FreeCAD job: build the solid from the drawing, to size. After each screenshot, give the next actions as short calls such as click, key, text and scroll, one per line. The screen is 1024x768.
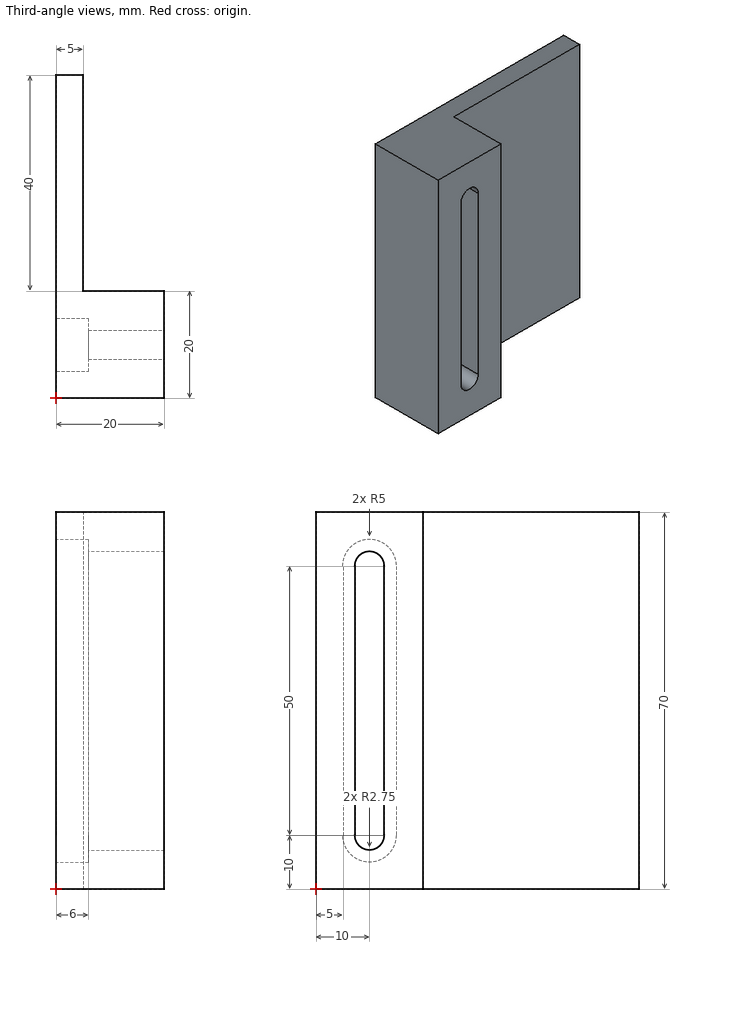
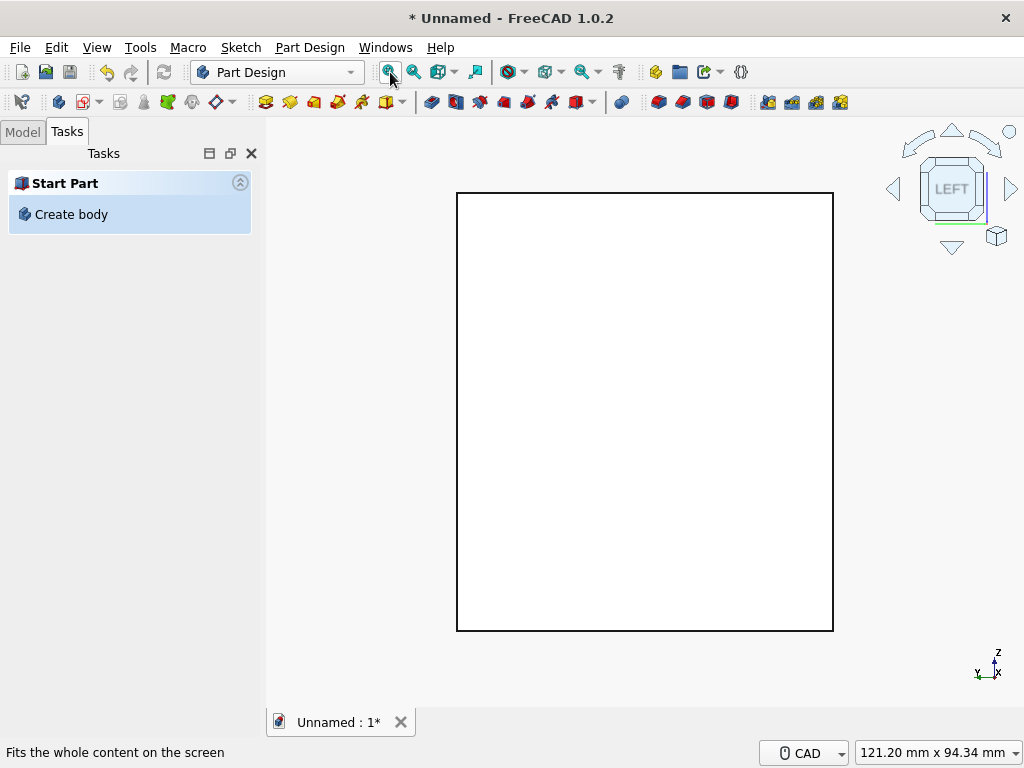
click(645, 411)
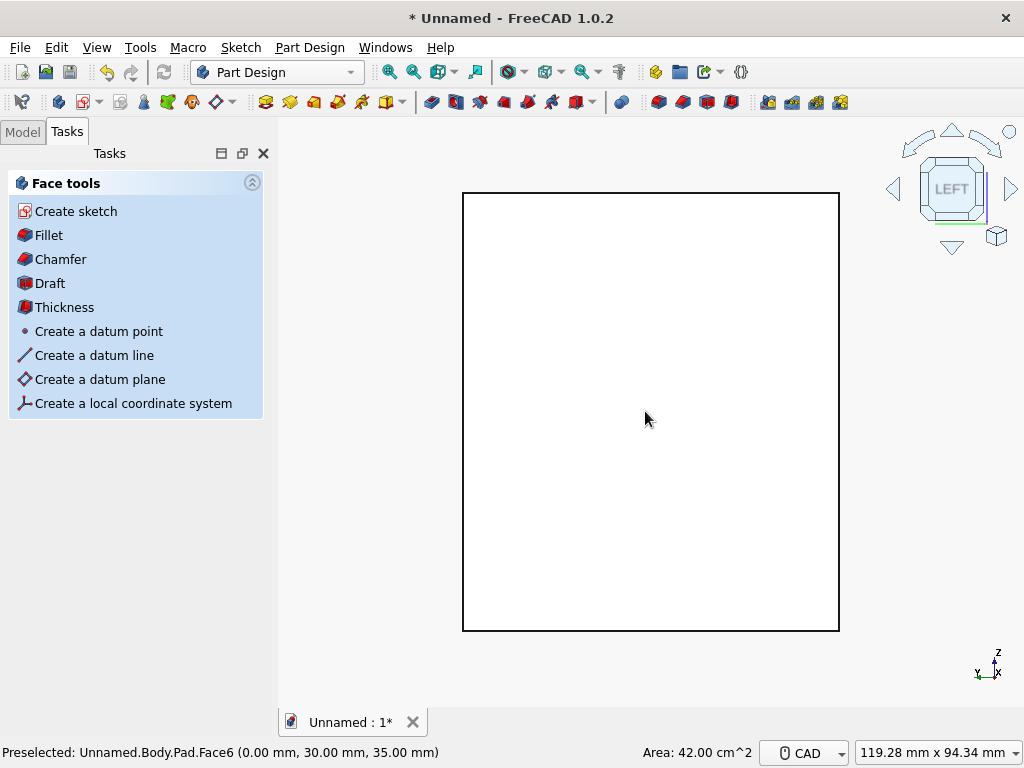
click(84, 102)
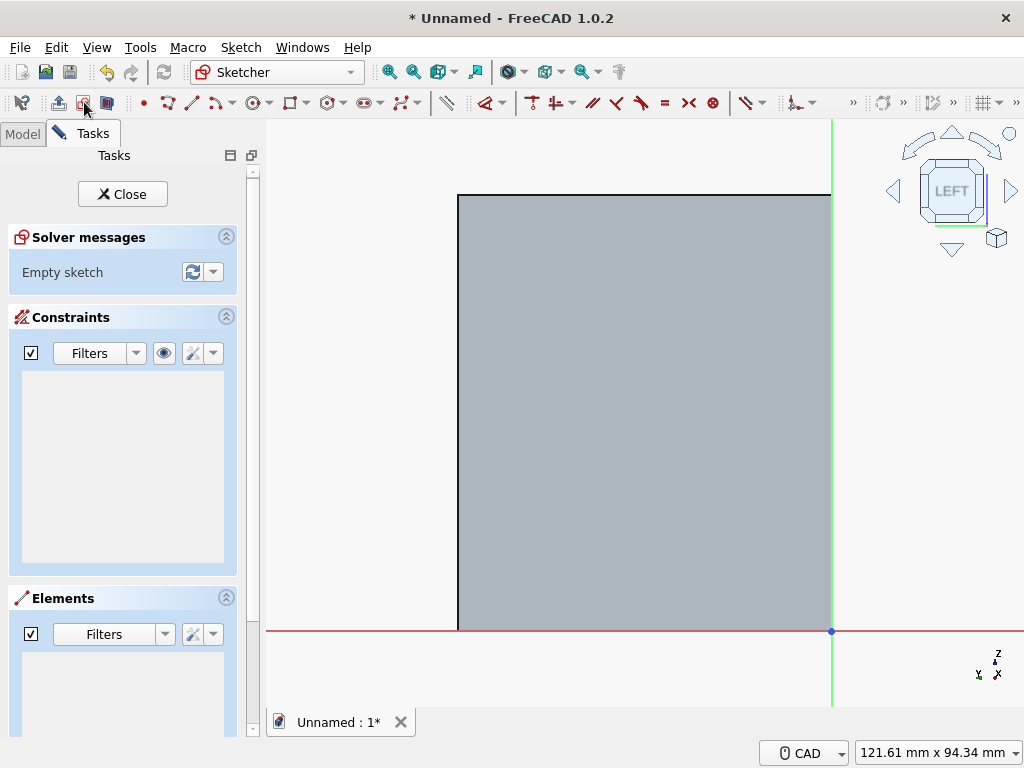
click(364, 104)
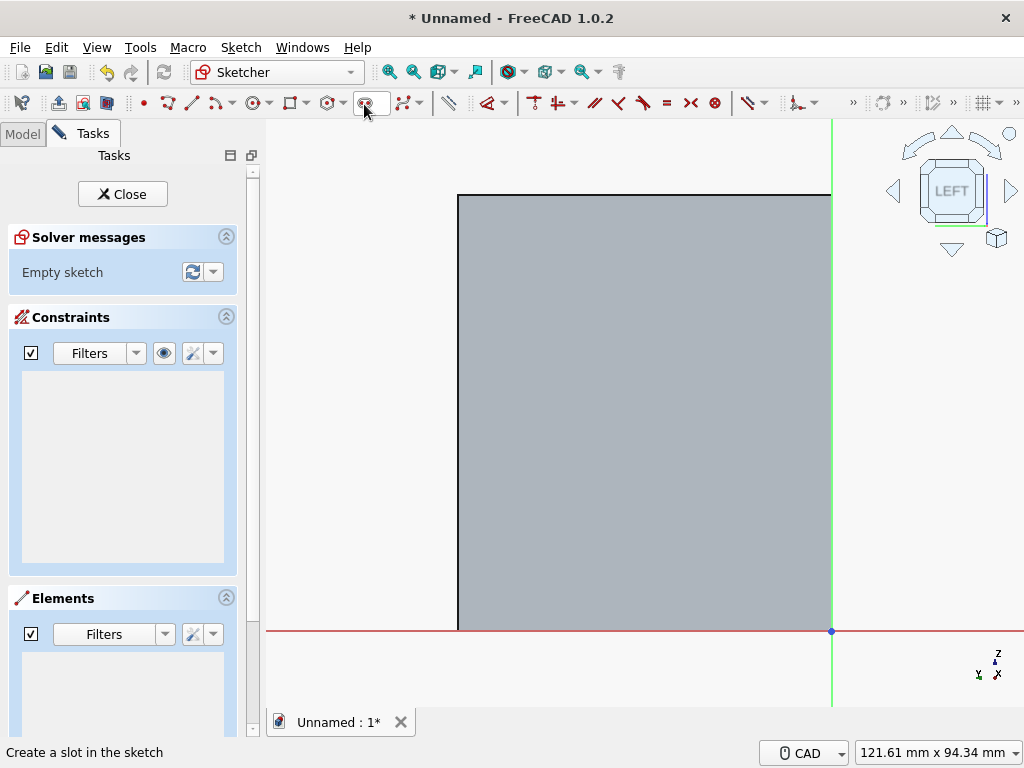
scroll(770, 569, up, 2)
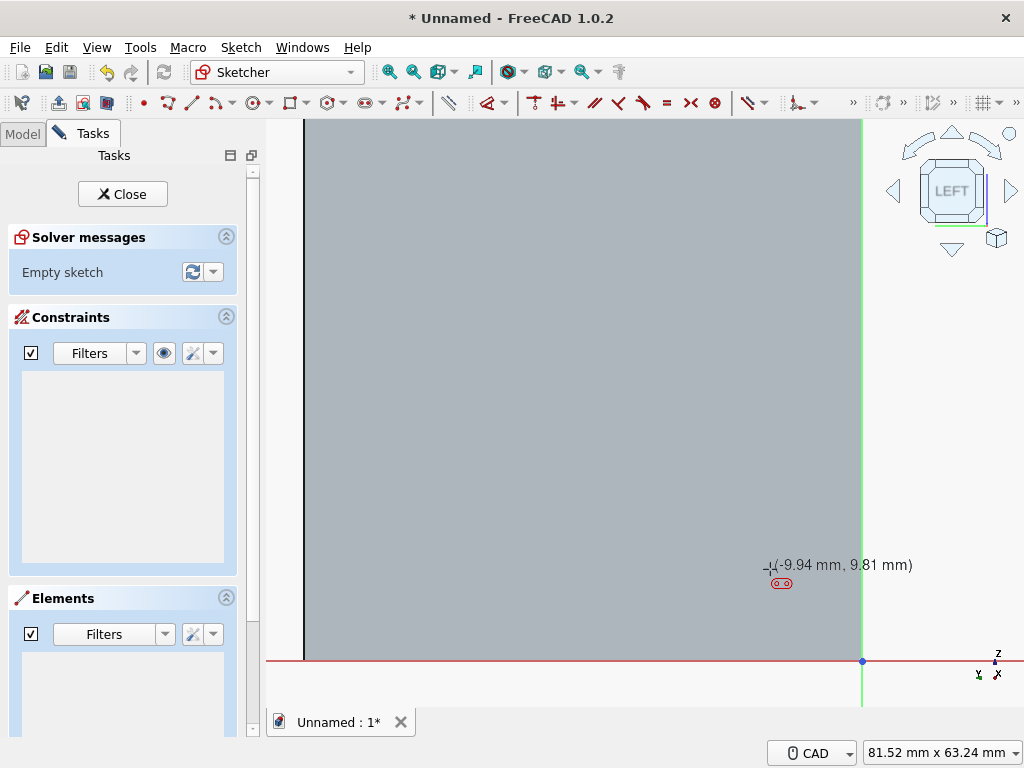
click(769, 568)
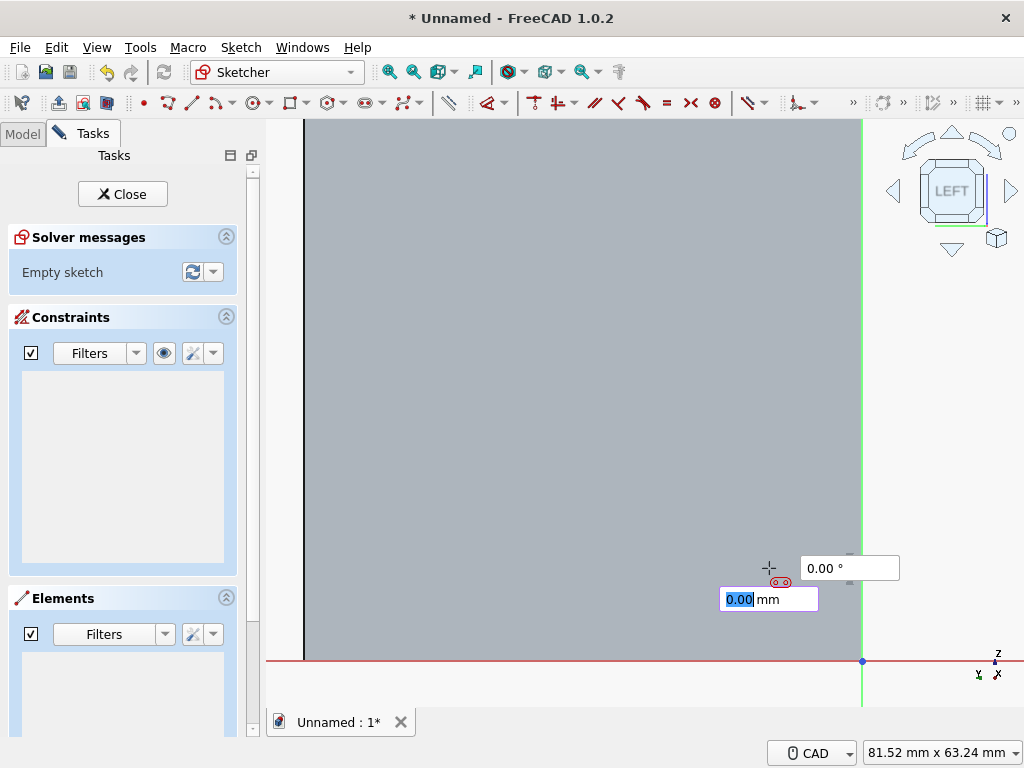
scroll(294, 501, down, 2)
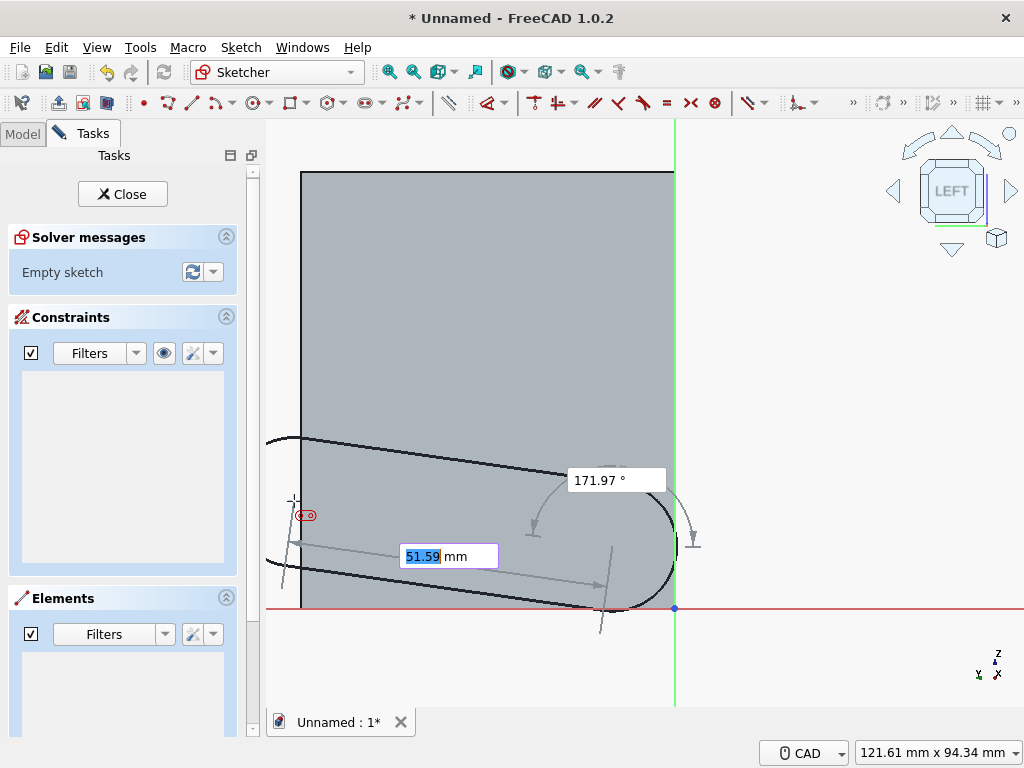
click(612, 235)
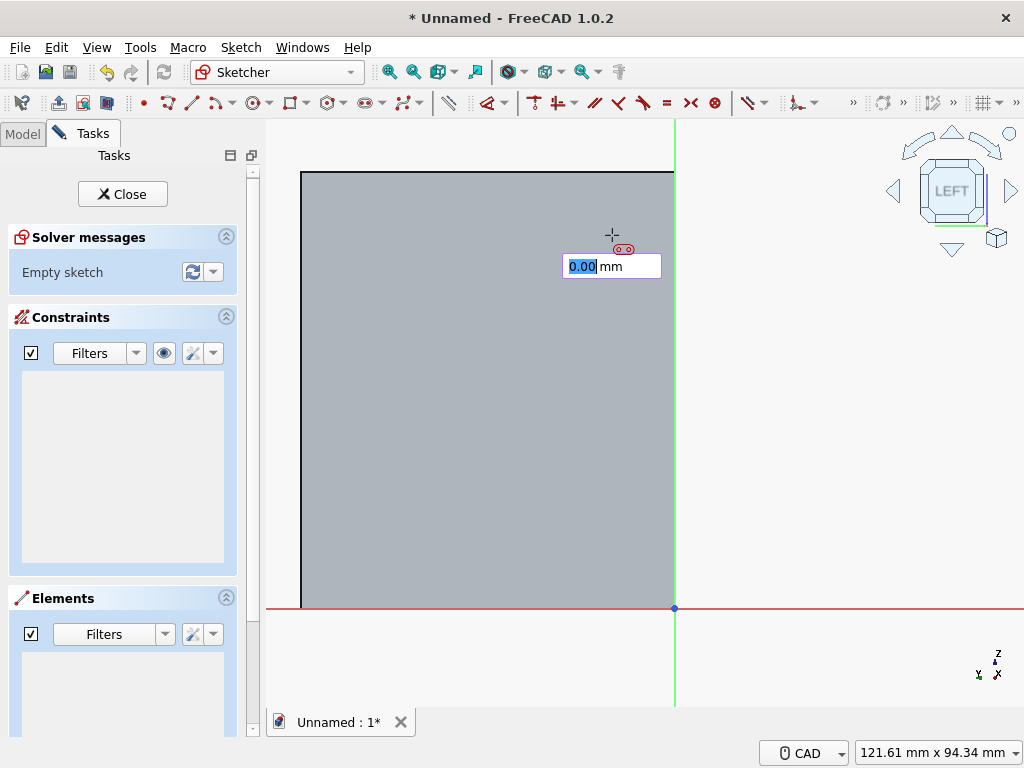
click(595, 391)
key(Escape)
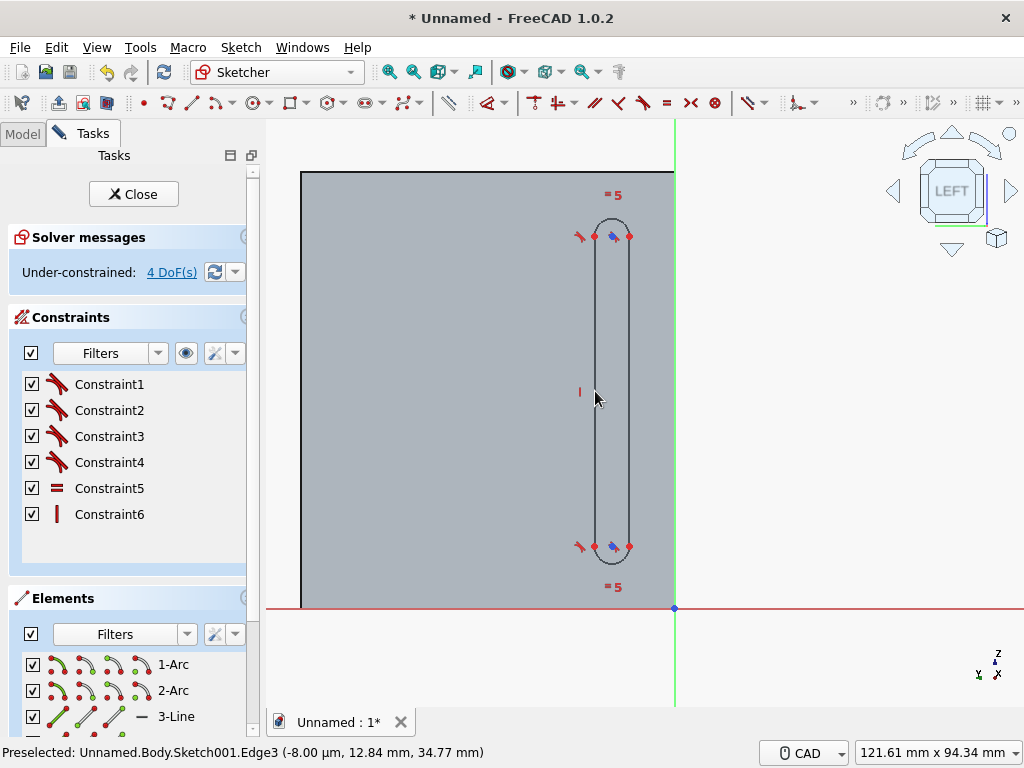
click(488, 104)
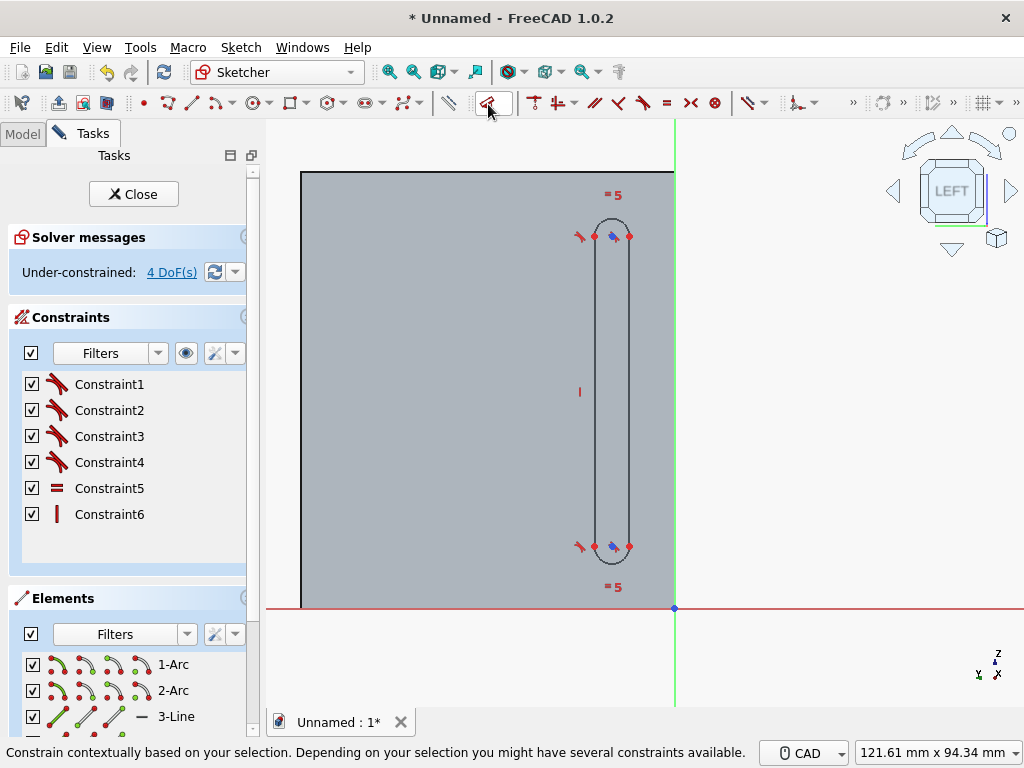
scroll(602, 561, up, 5)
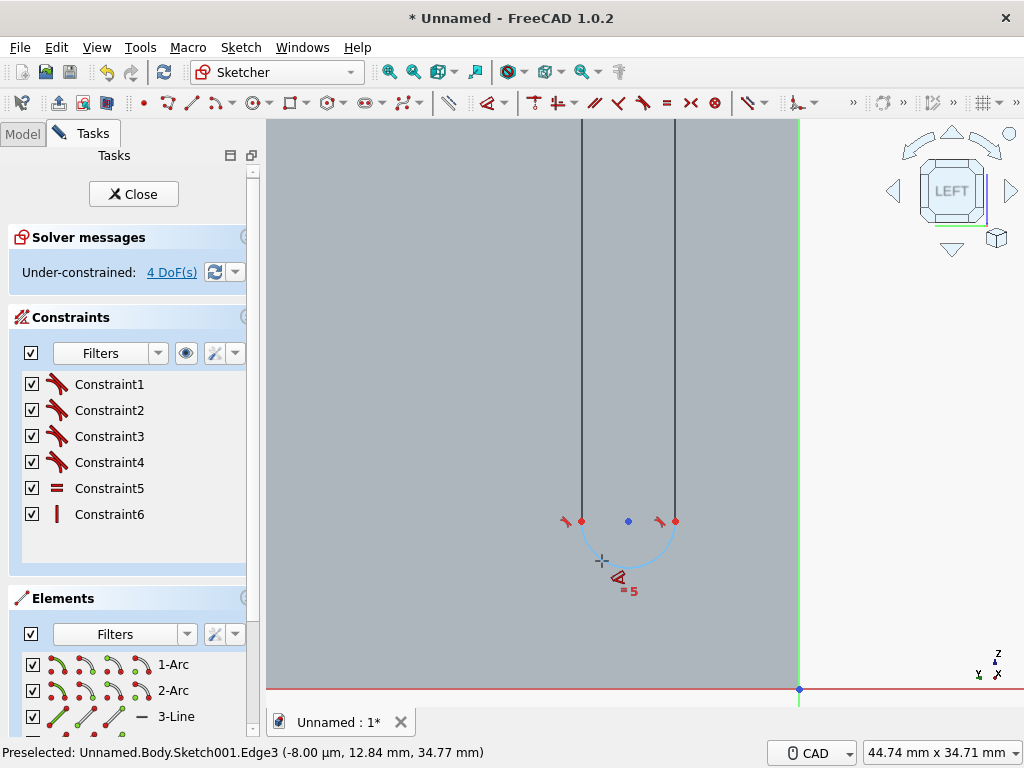
click(601, 559)
click(582, 585)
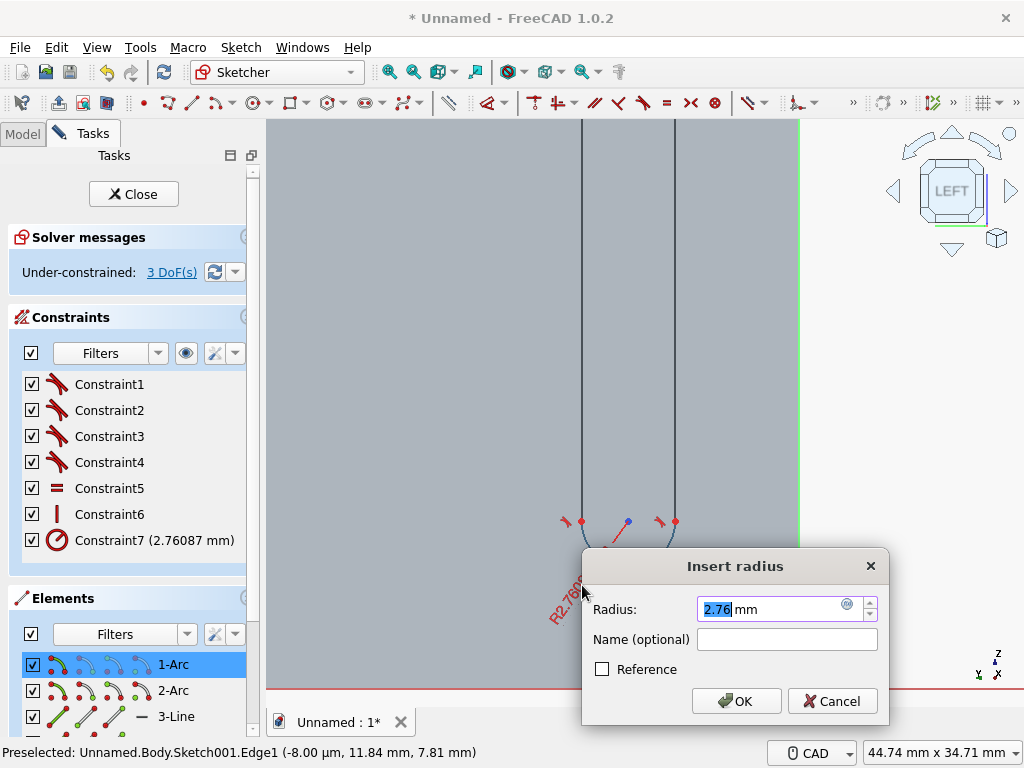
text(2.75)
key(Return)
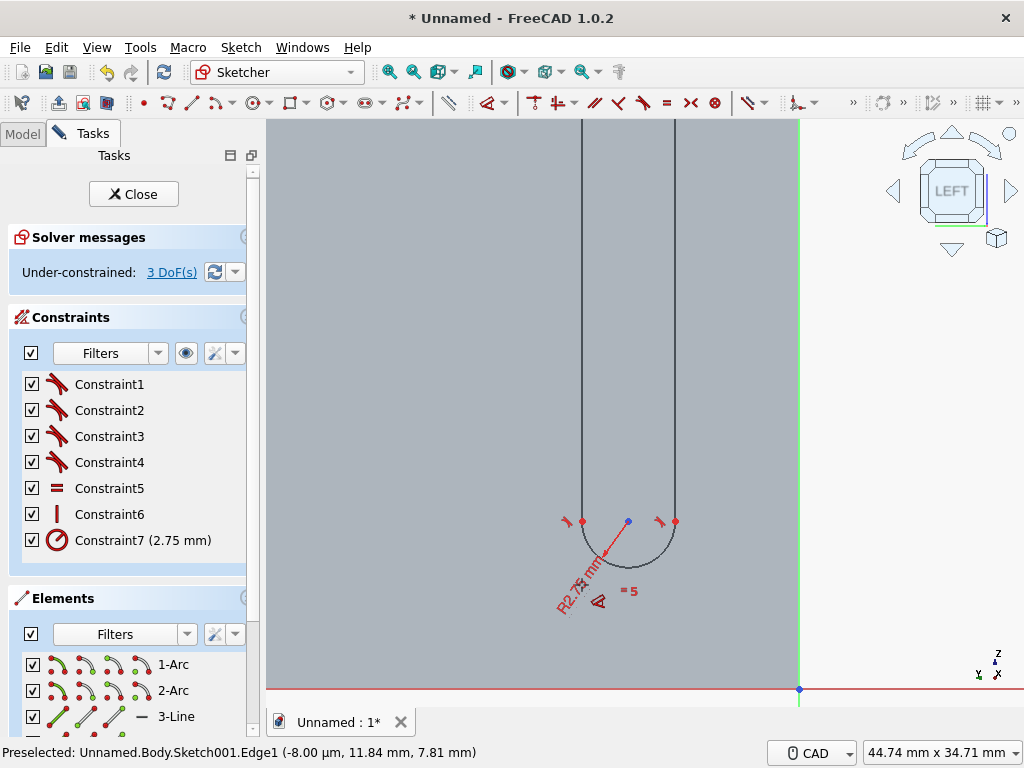
click(582, 268)
click(548, 334)